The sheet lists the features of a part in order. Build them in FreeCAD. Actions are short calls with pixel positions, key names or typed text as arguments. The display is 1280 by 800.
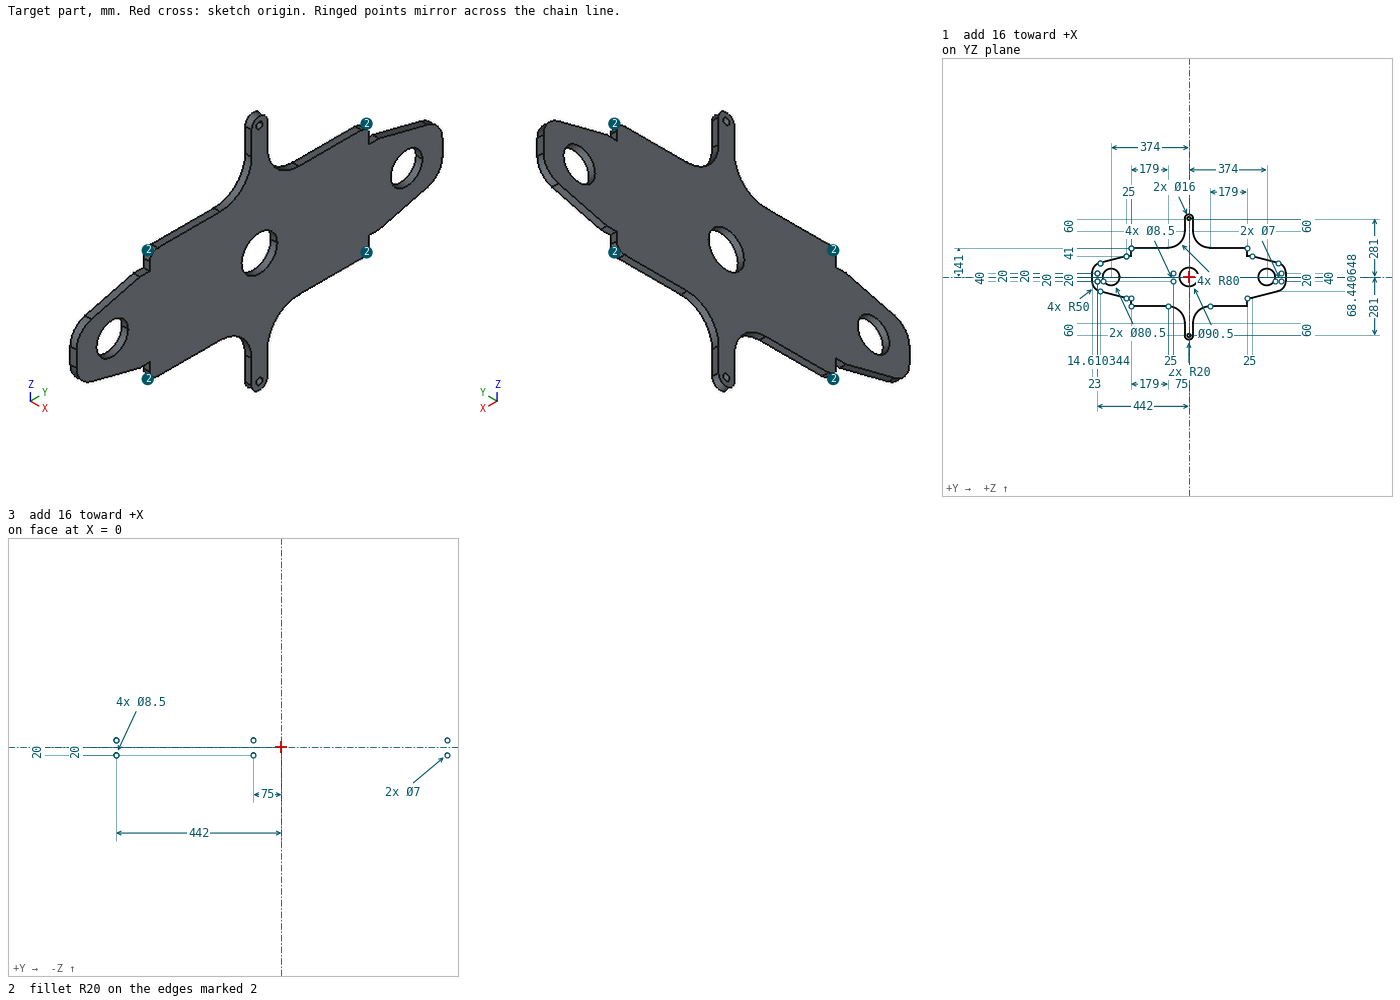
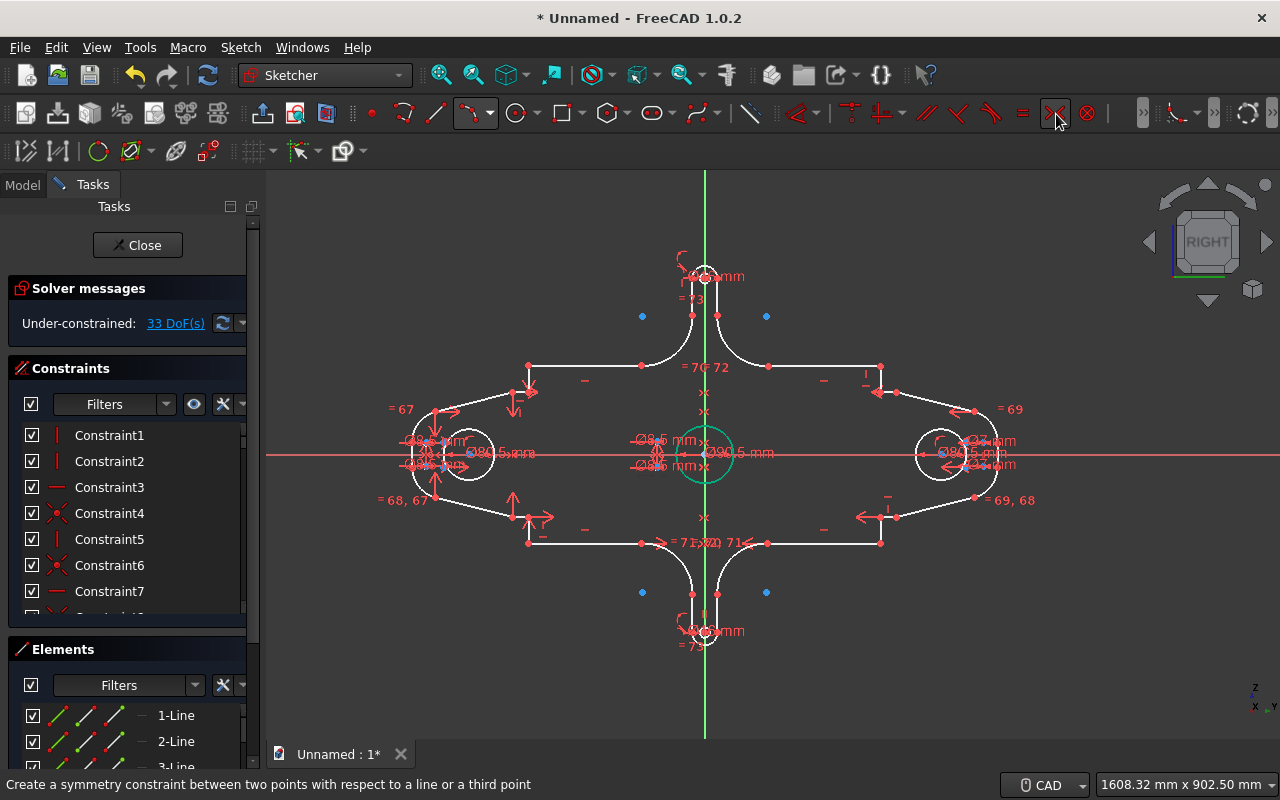
click(529, 366)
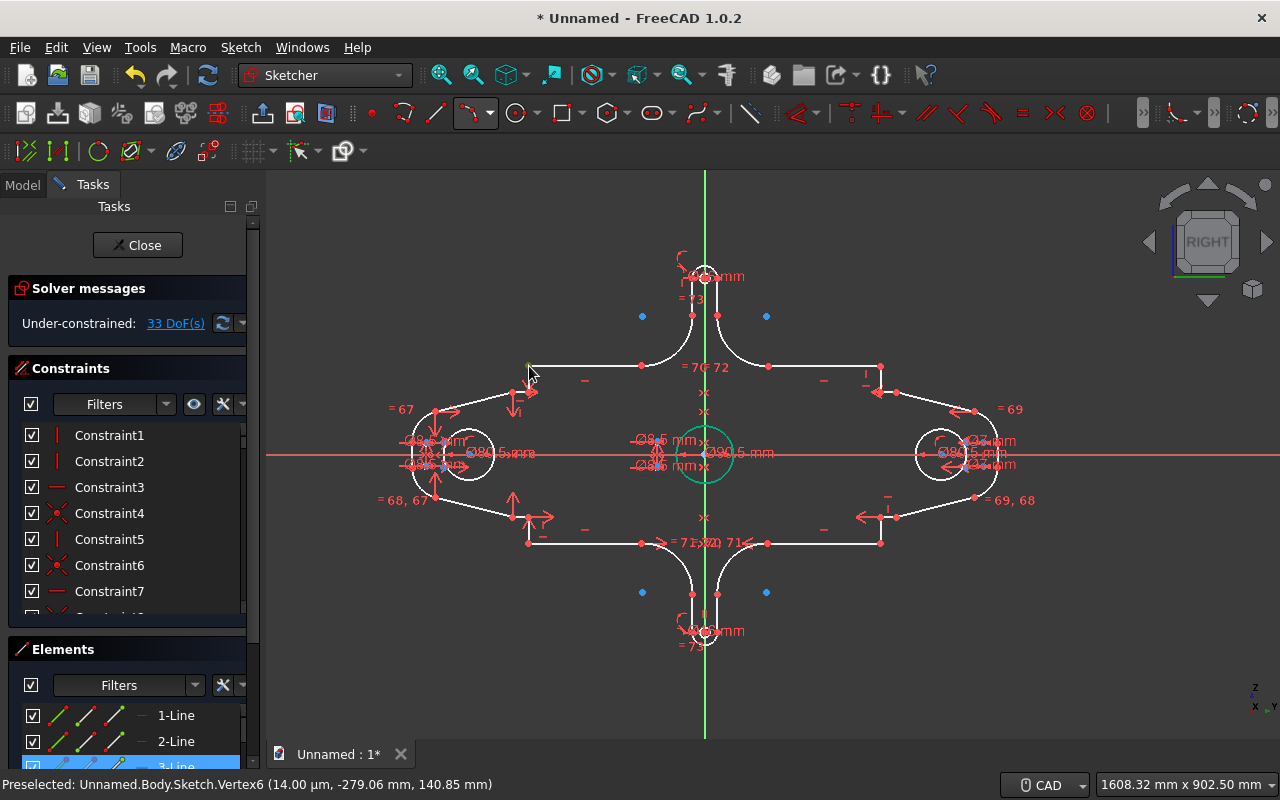
click(881, 366)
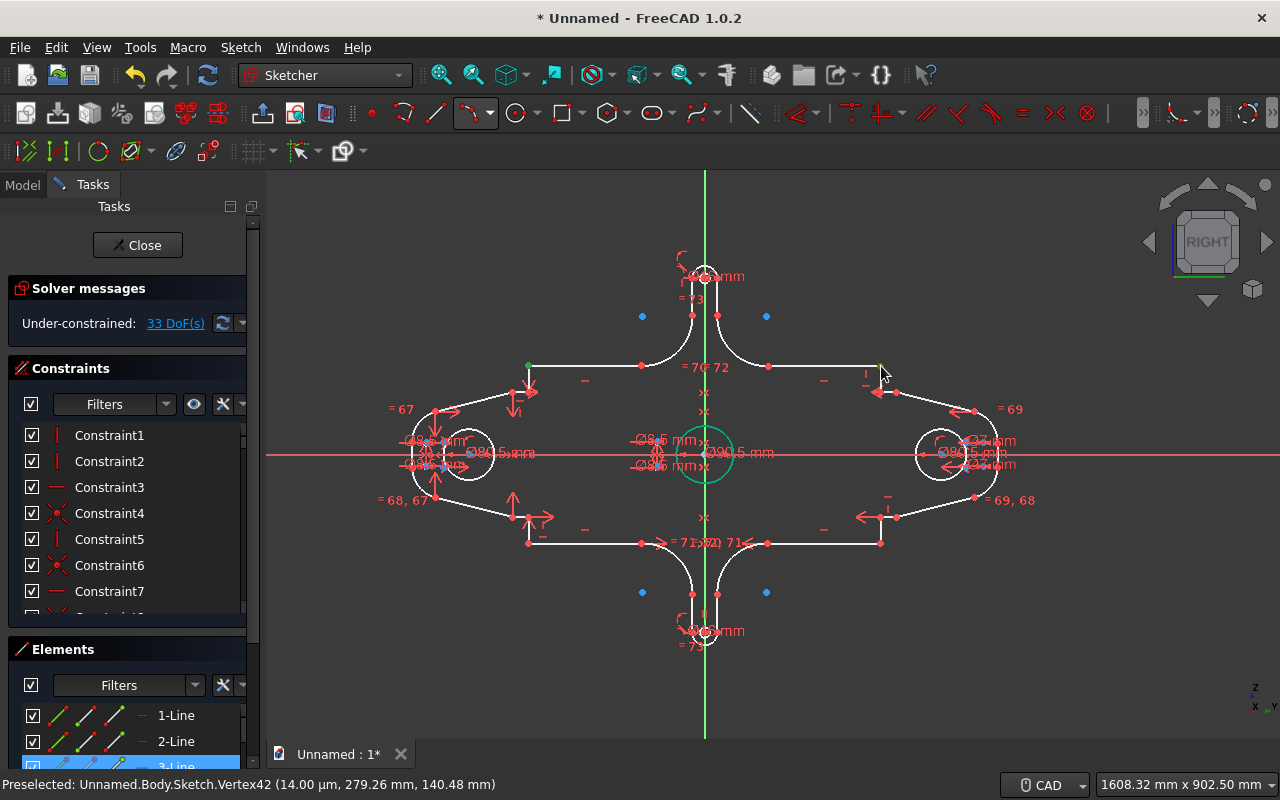
click(705, 528)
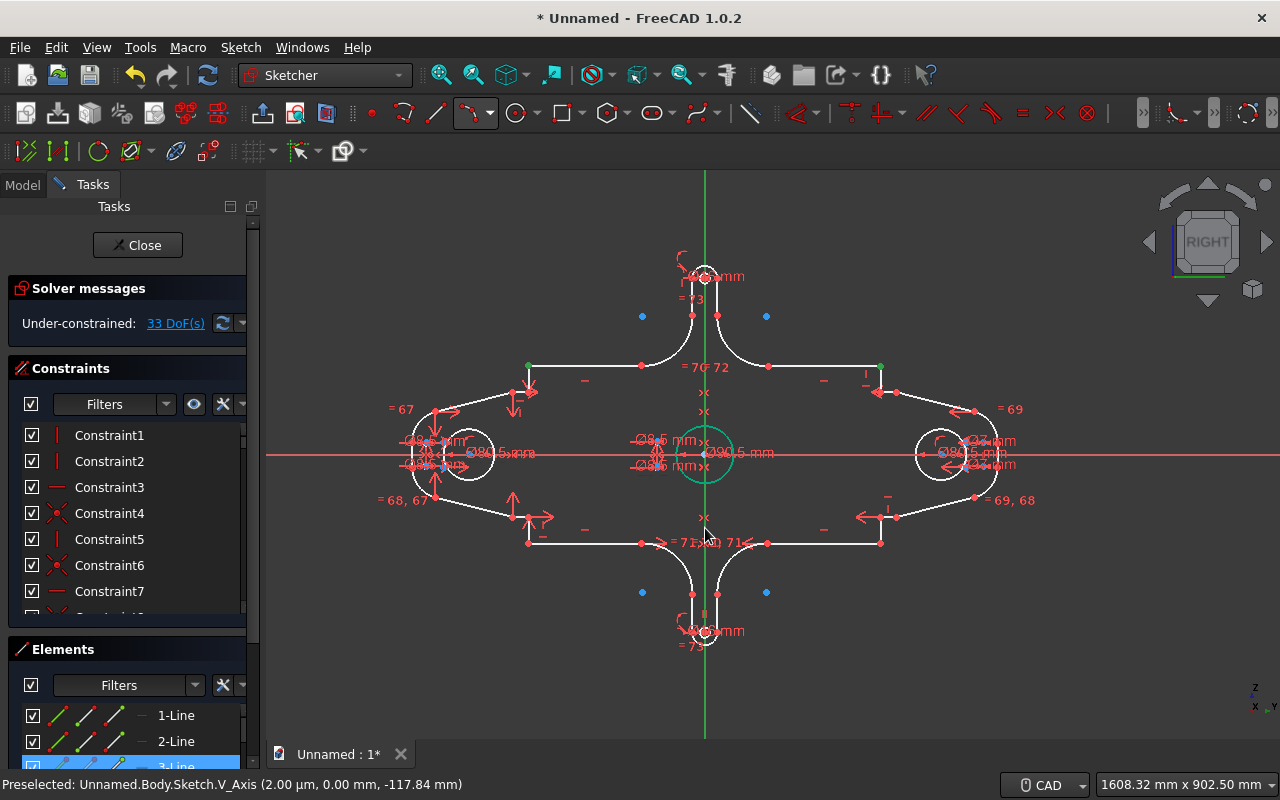
key(s)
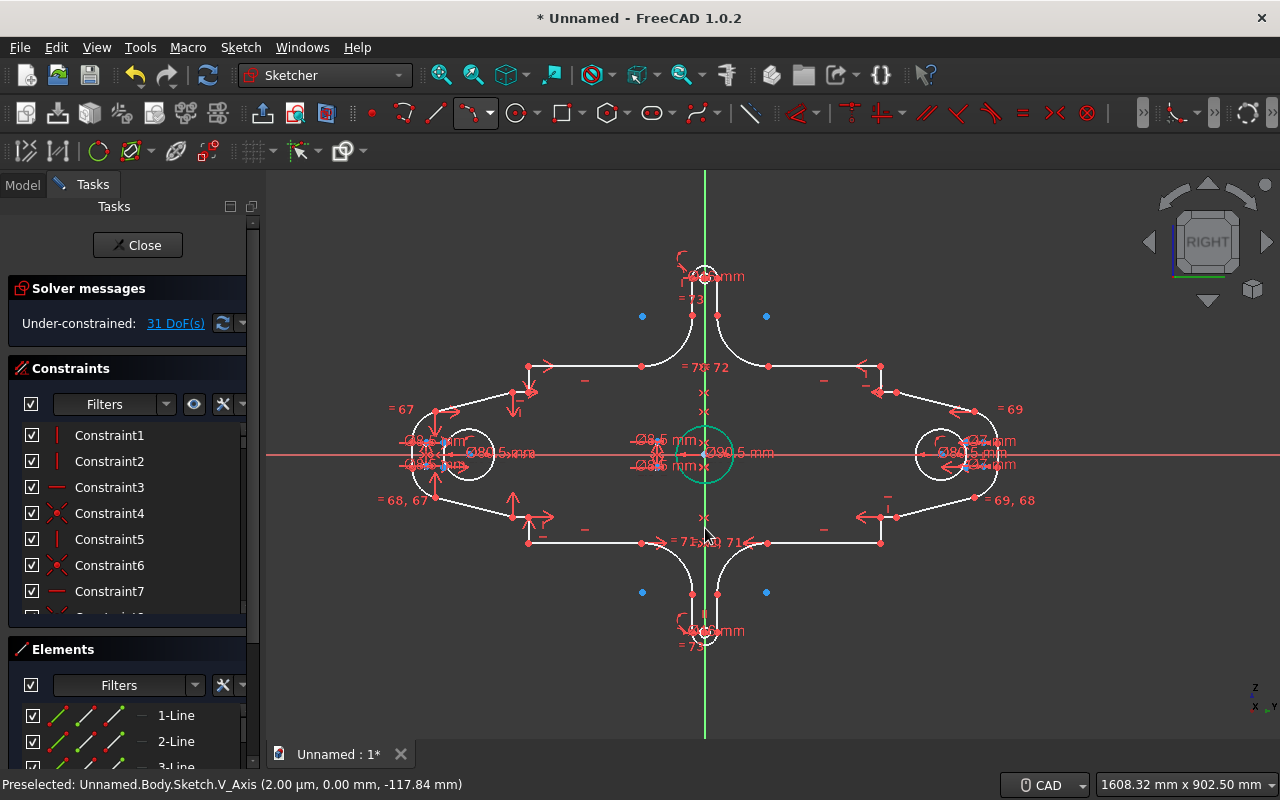
scroll(715, 271, up, 6)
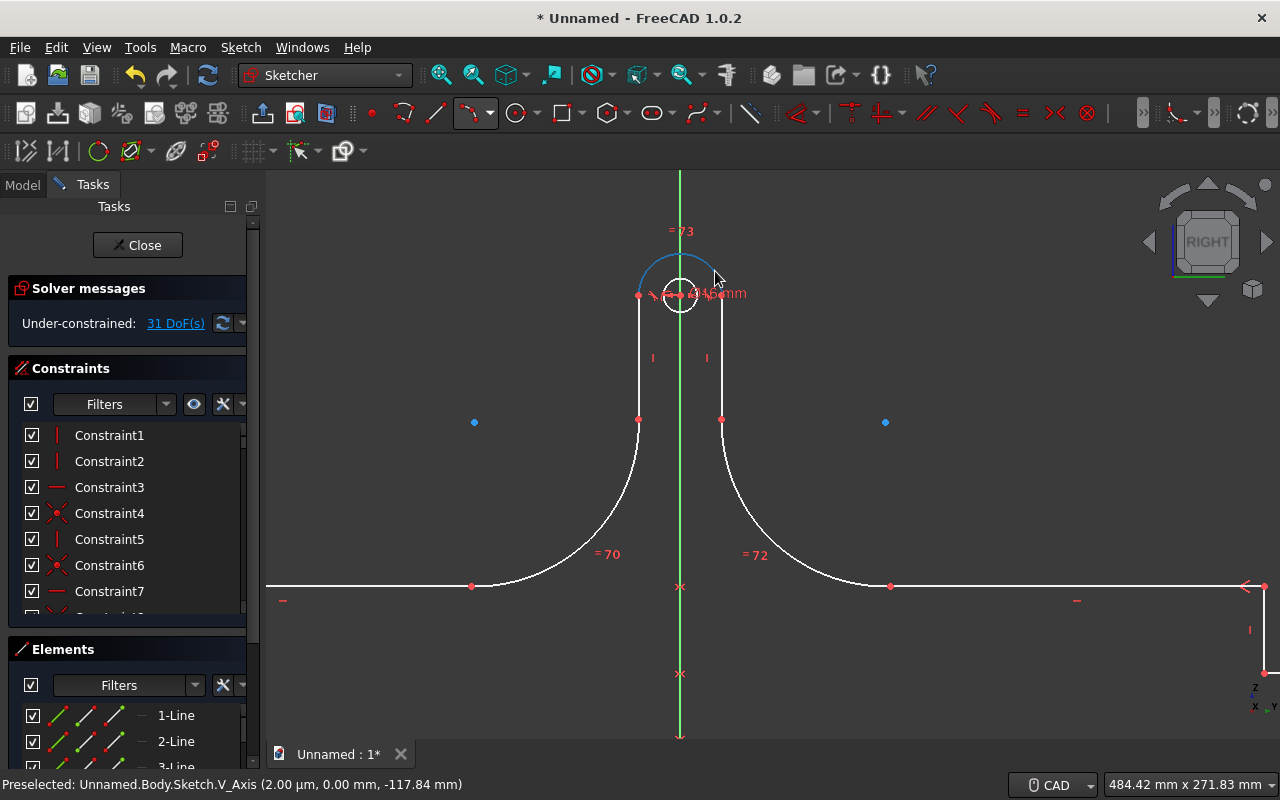
click(714, 271)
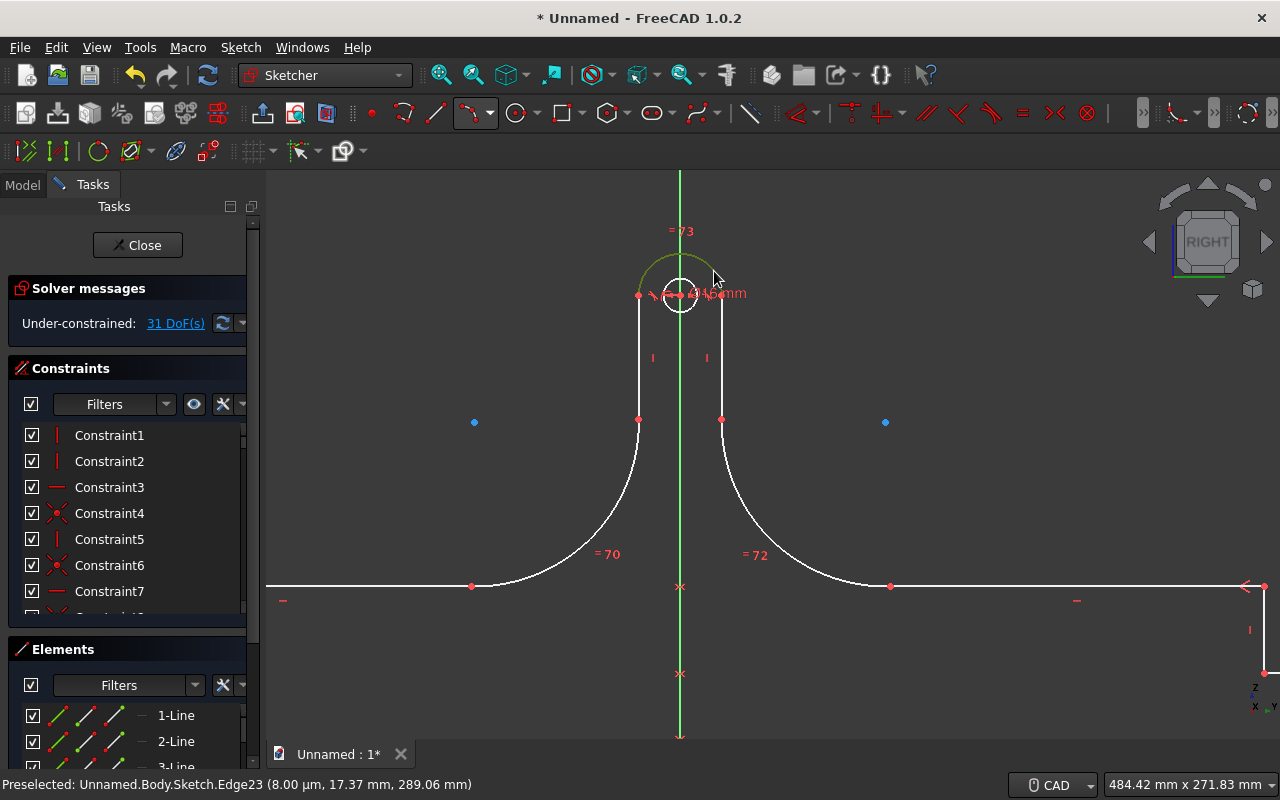
click(818, 114)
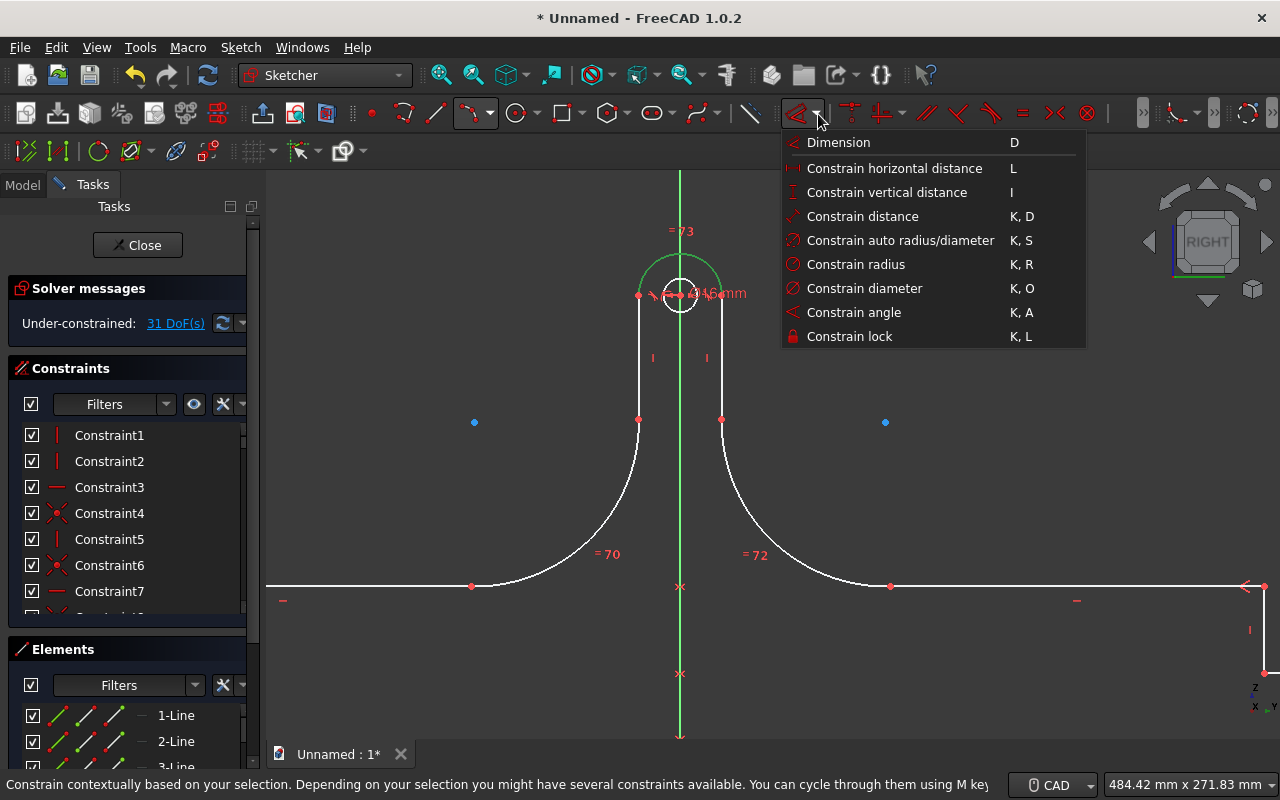
click(934, 264)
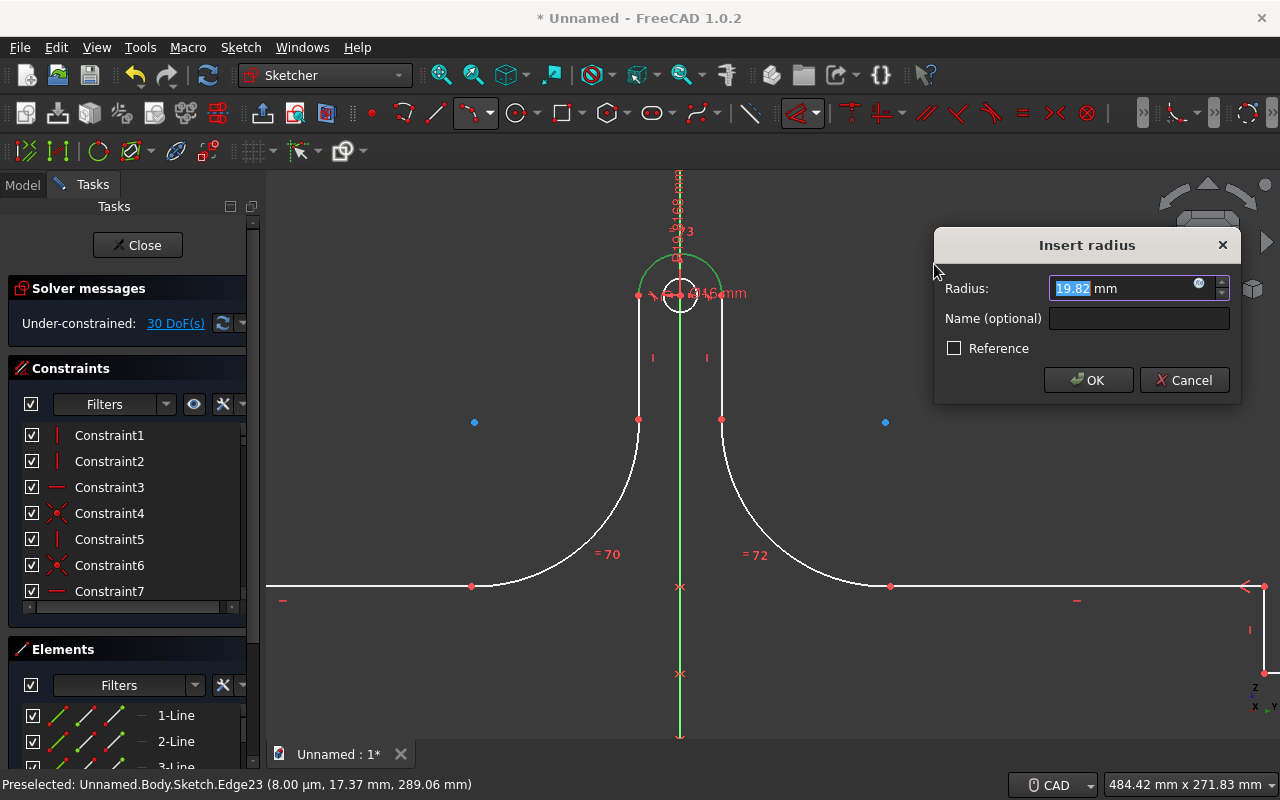
text(20)
key(Return)